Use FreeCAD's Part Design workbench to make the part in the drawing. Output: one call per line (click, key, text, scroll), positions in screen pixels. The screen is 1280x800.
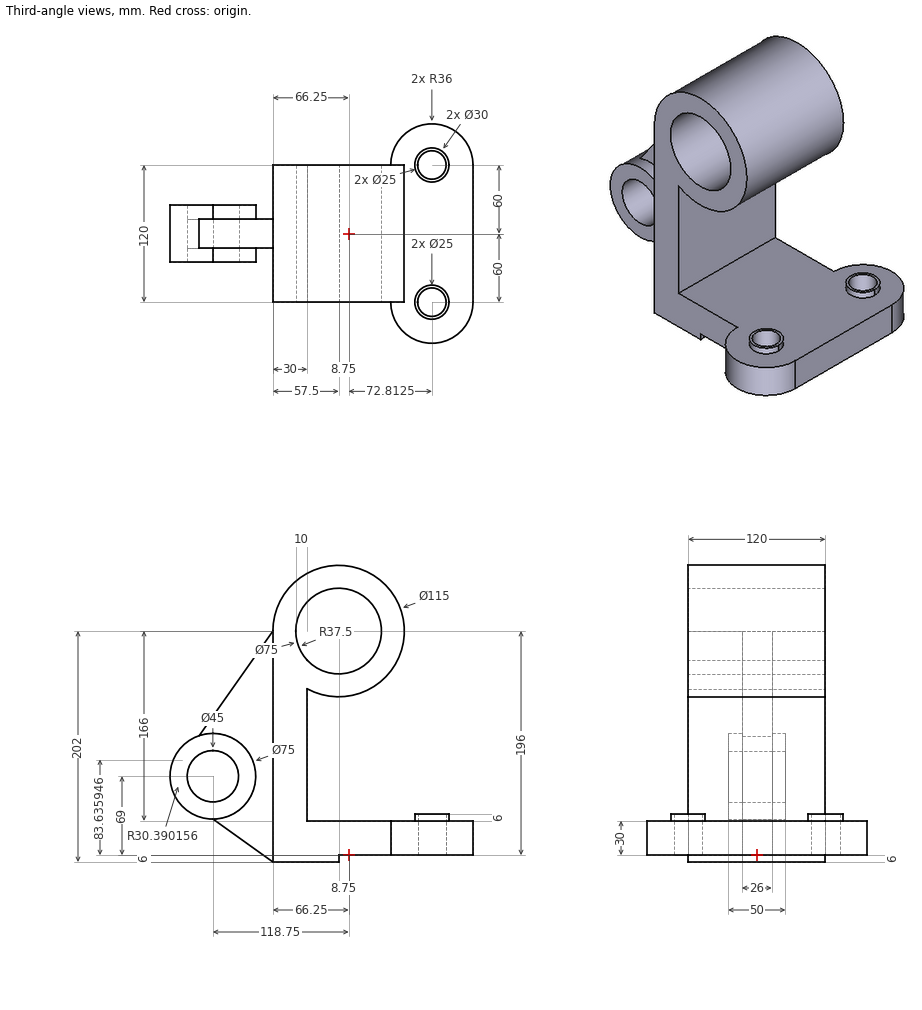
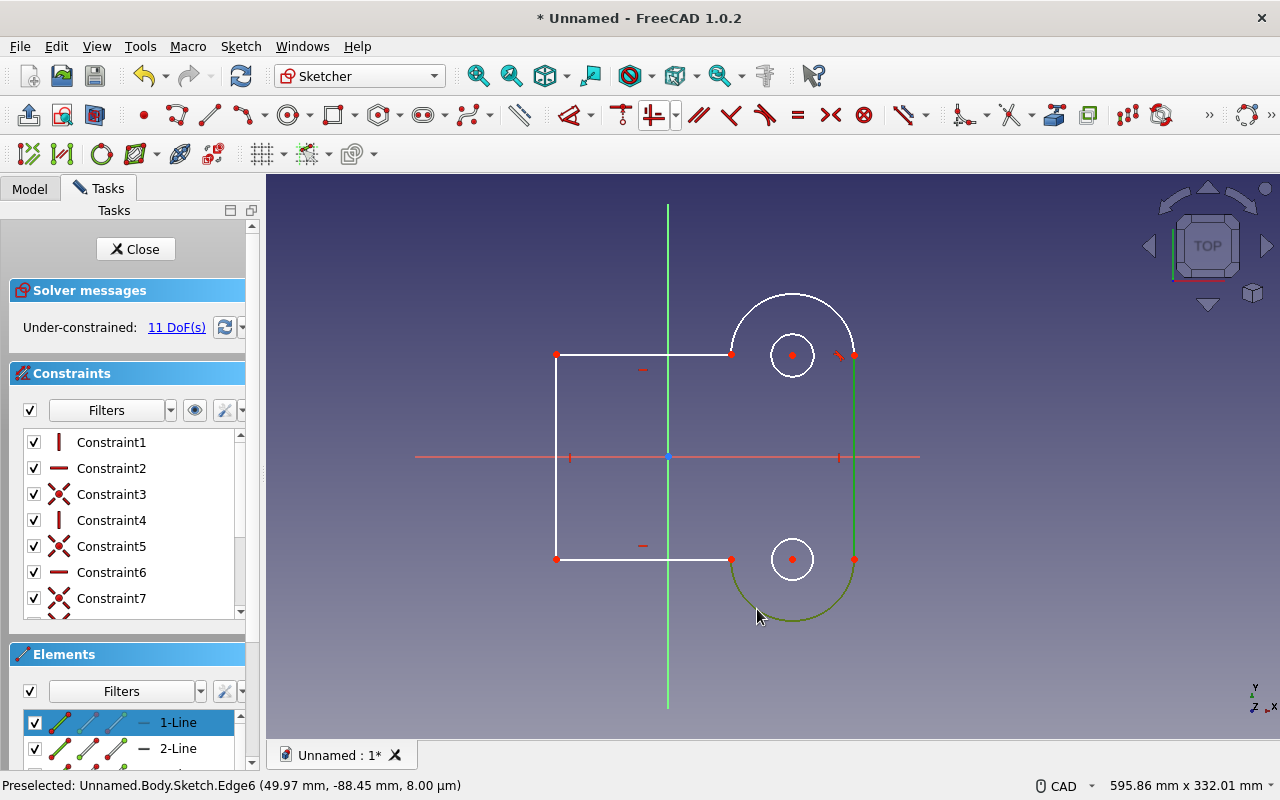
key(t)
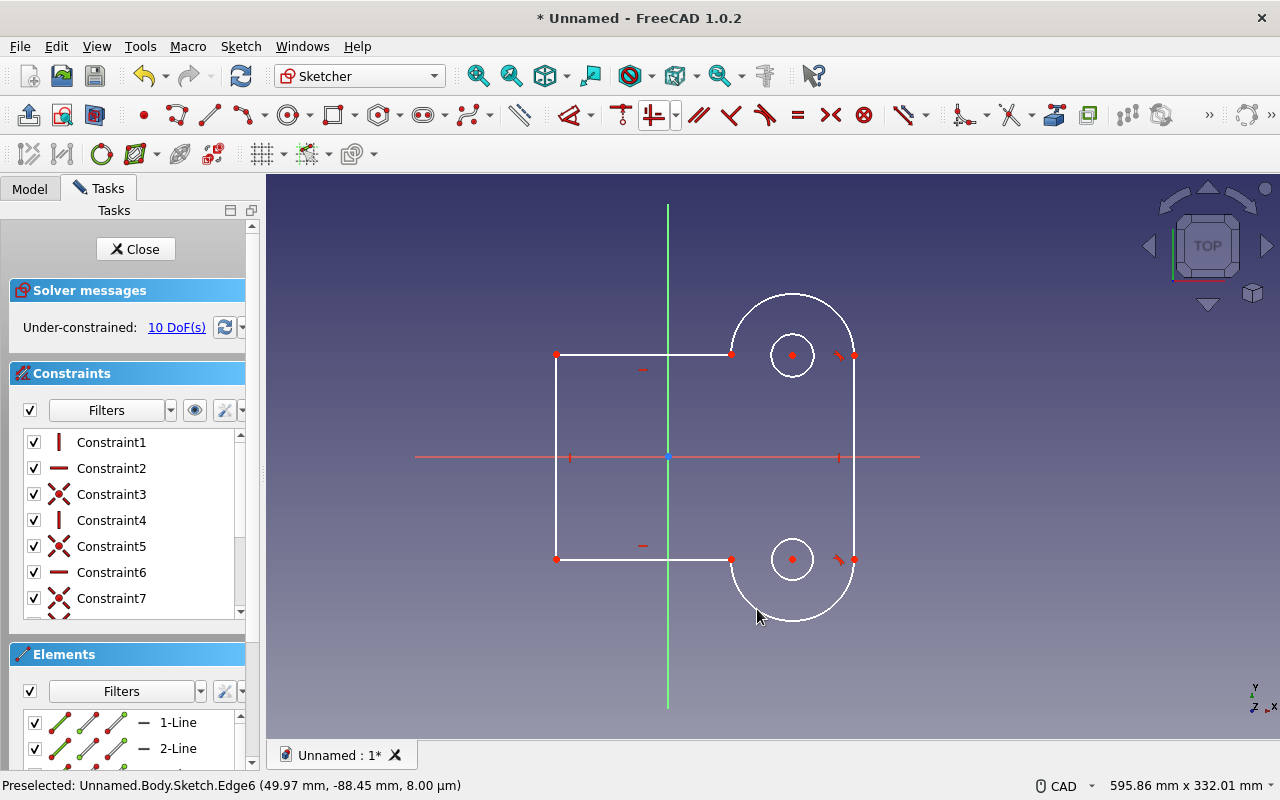
click(829, 306)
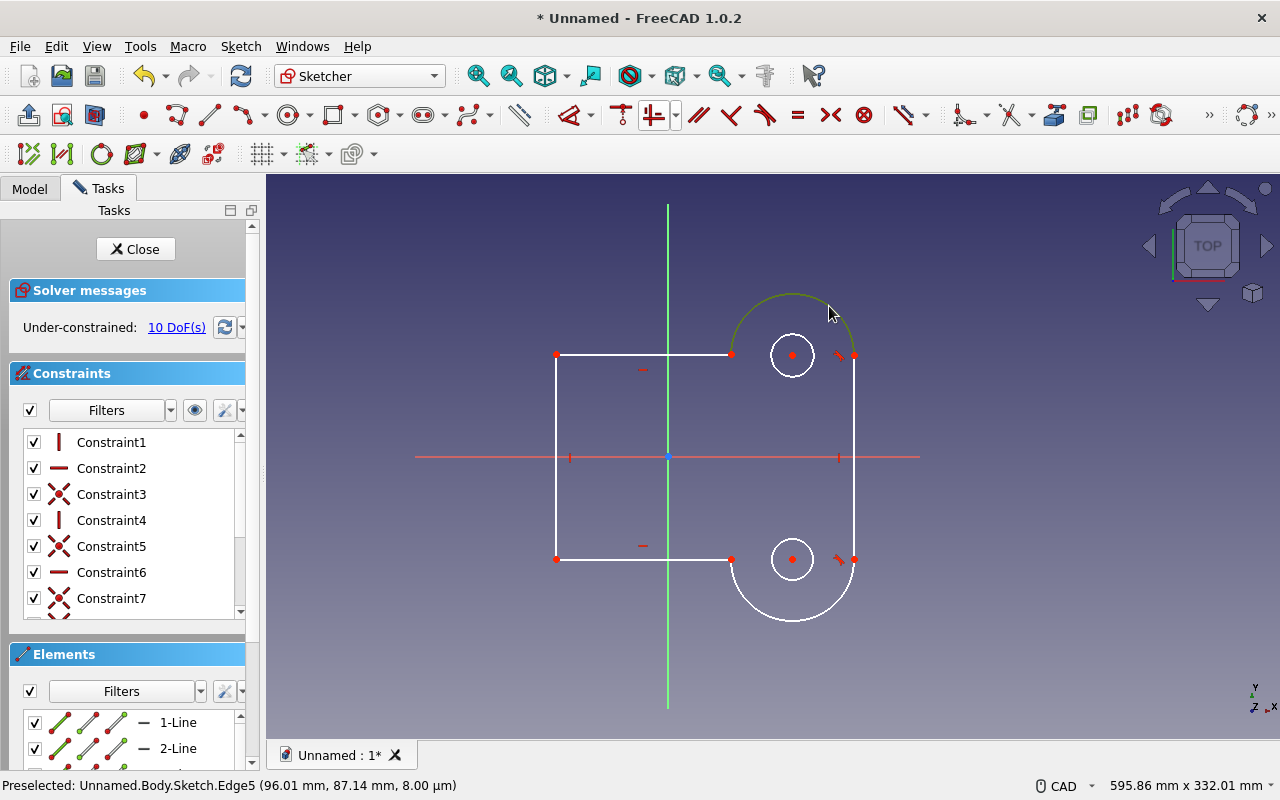
click(757, 609)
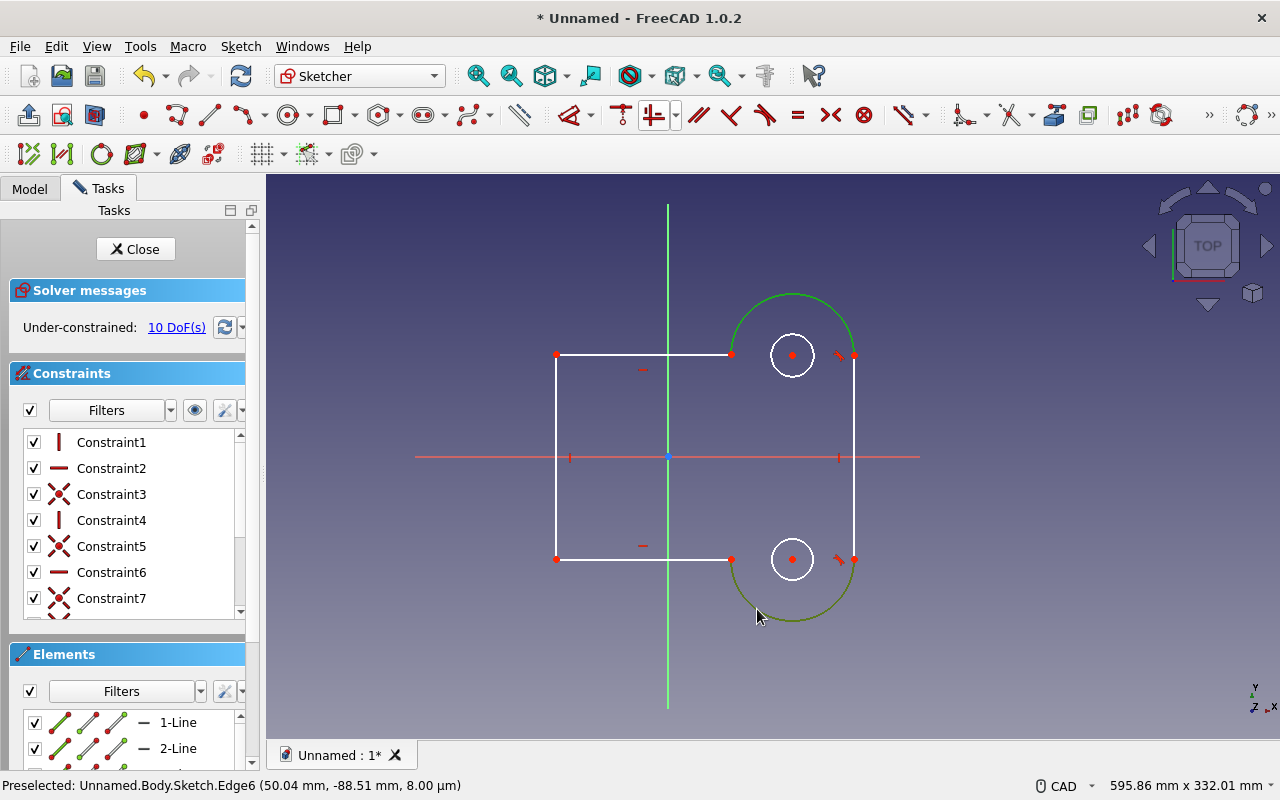
key(e)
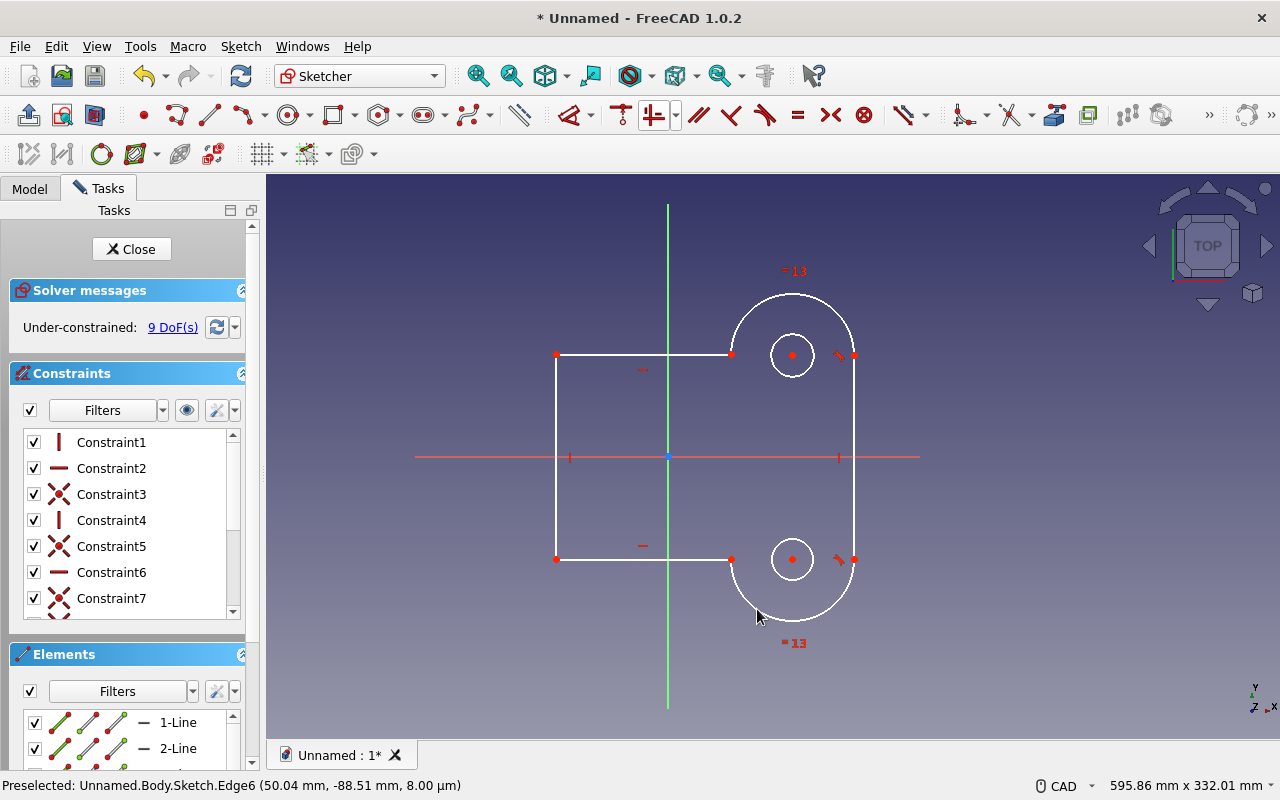
click(807, 545)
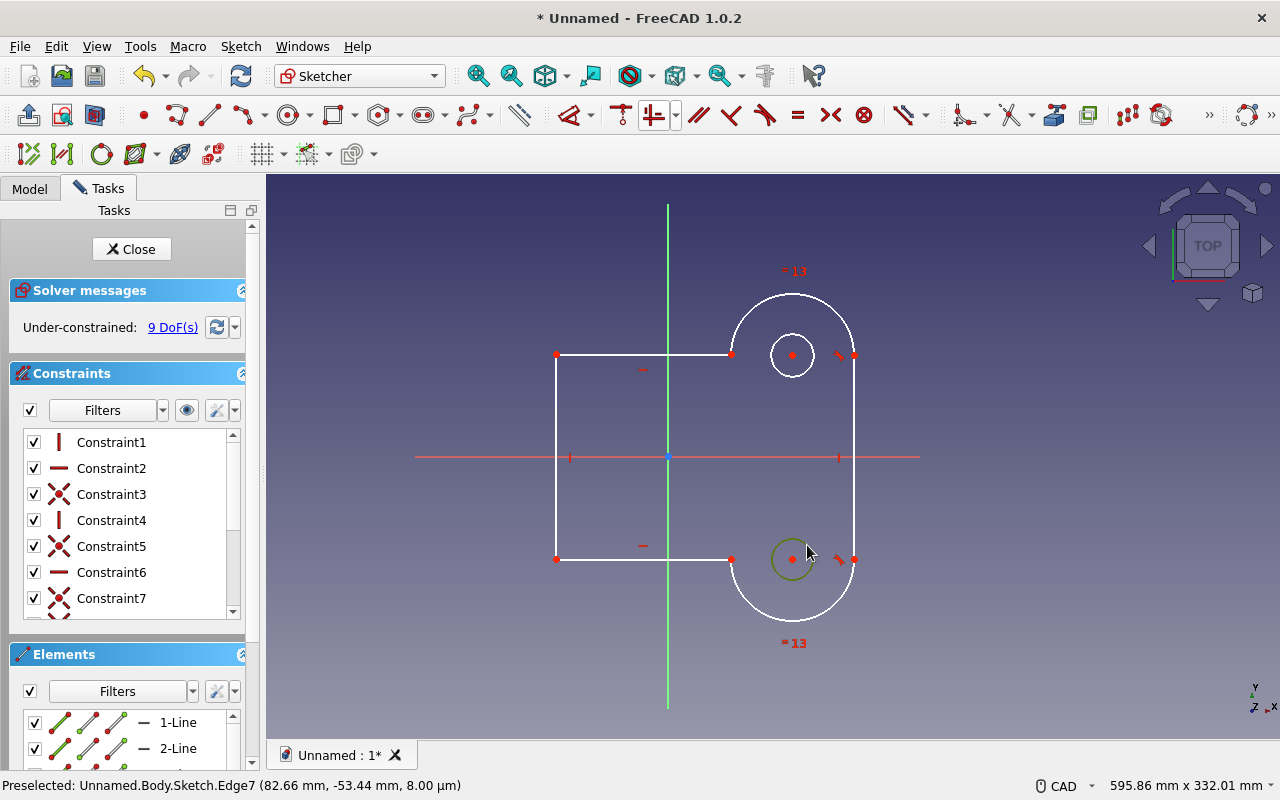
click(807, 340)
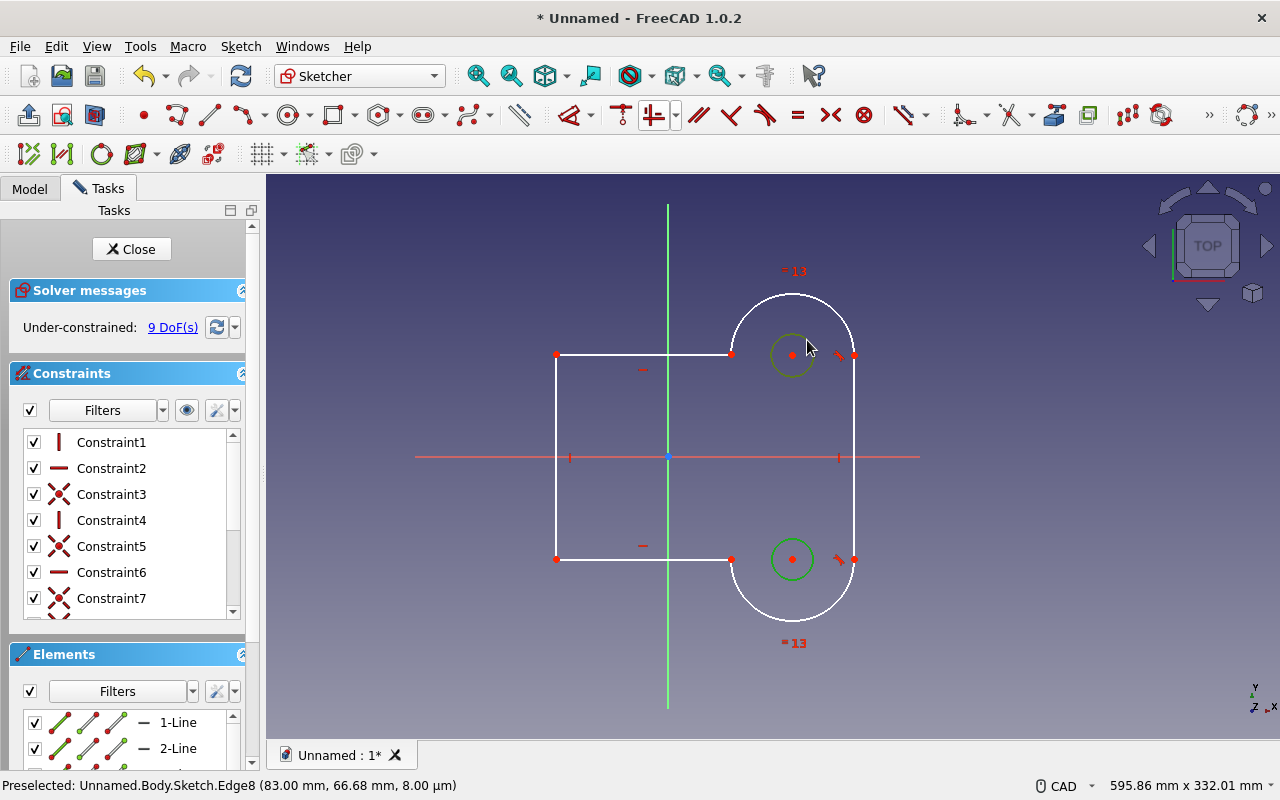
key(e)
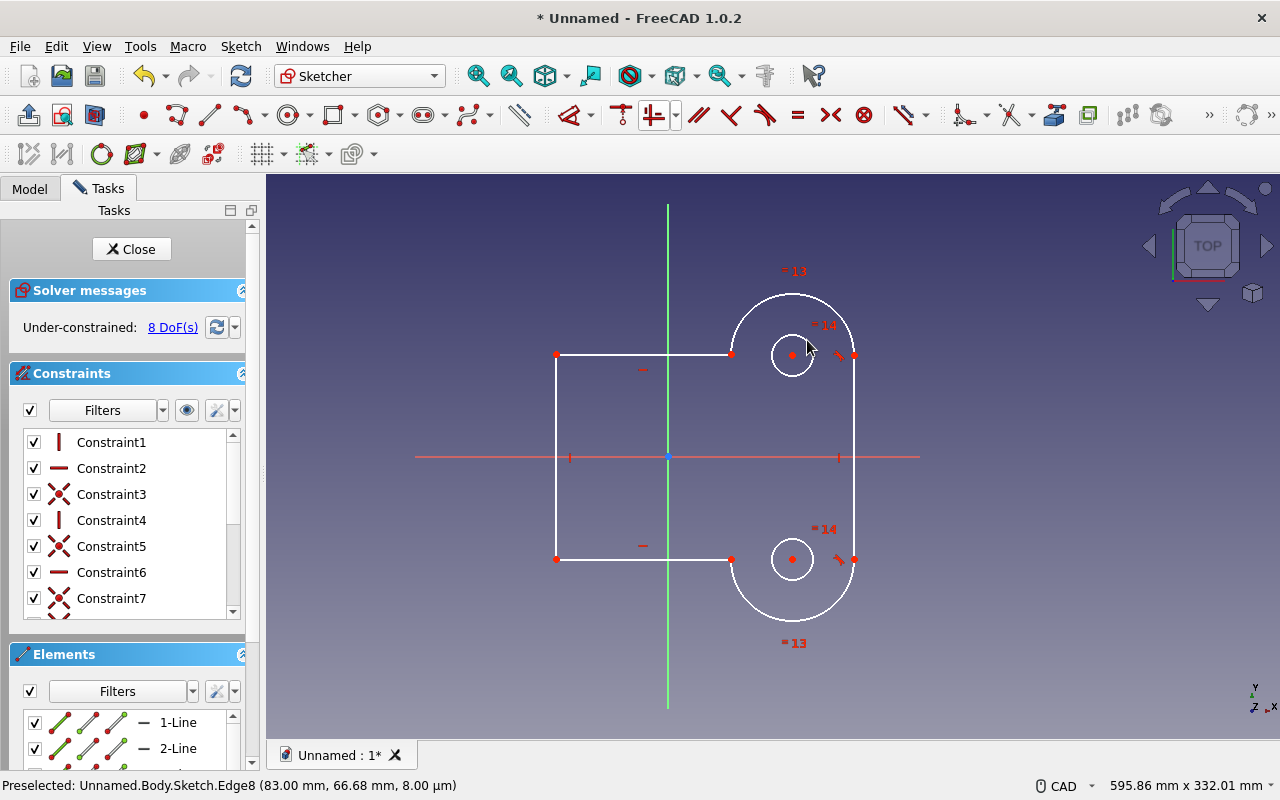
click(829, 306)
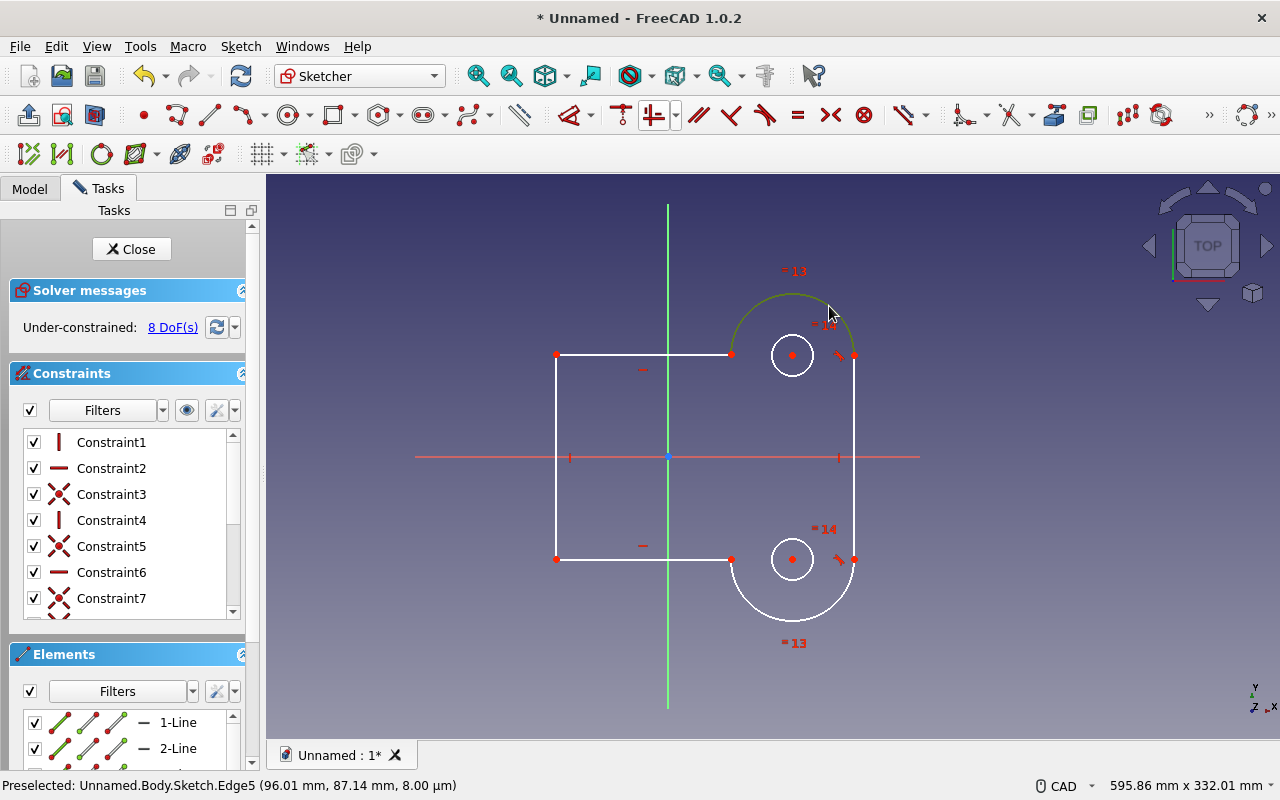
click(590, 116)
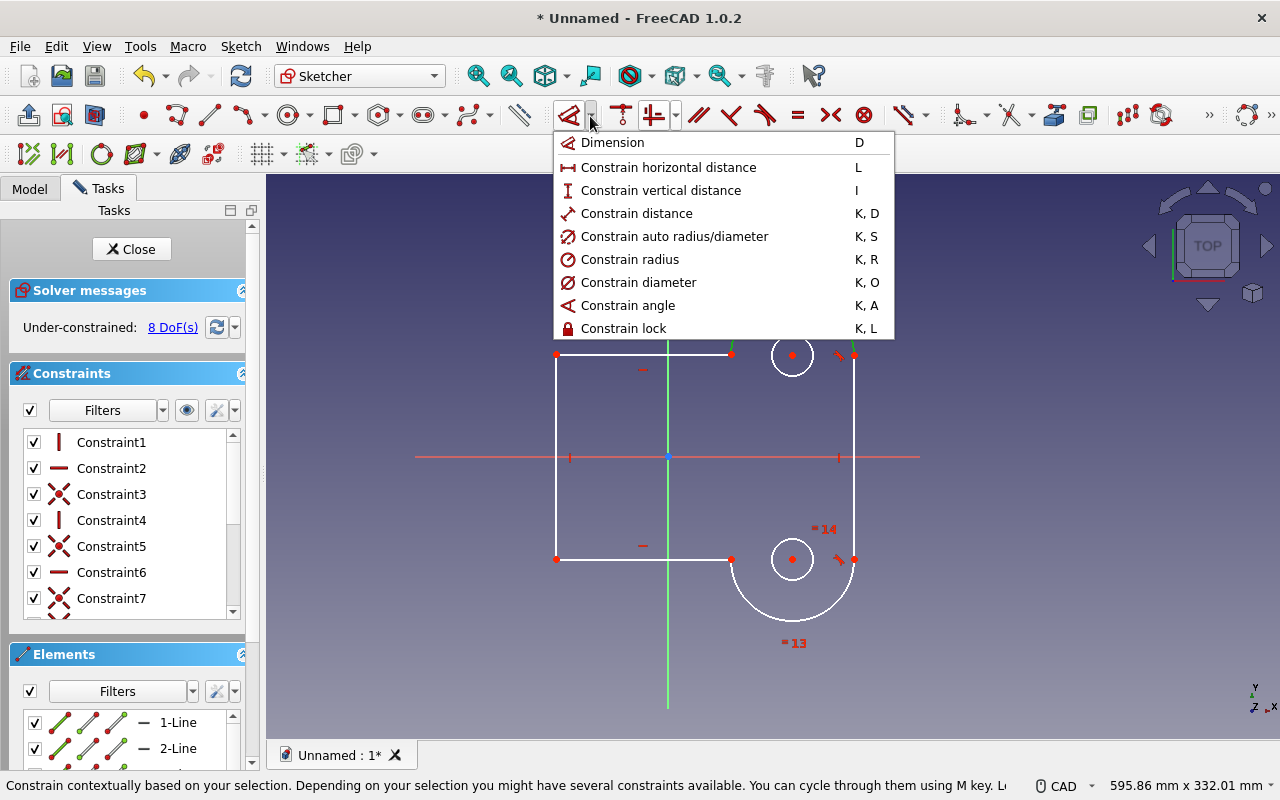
click(724, 260)